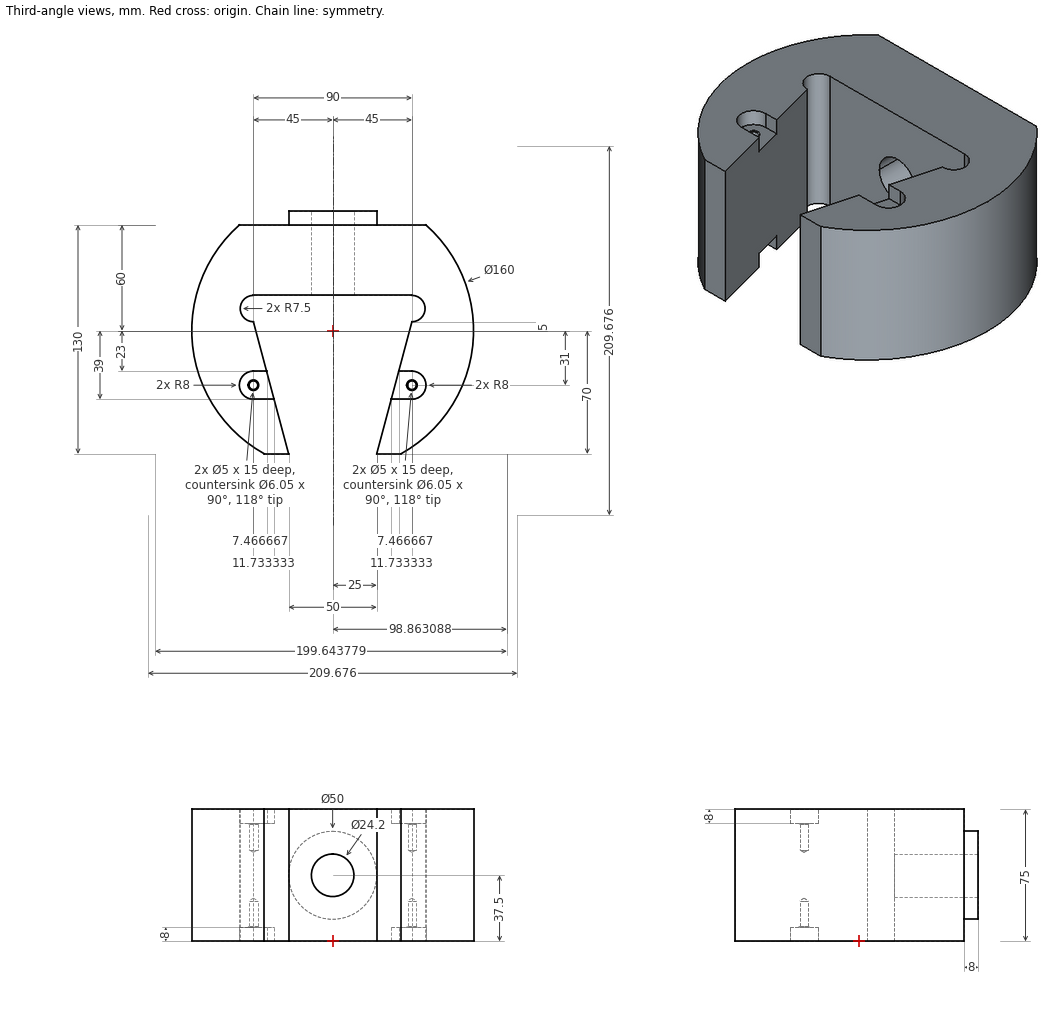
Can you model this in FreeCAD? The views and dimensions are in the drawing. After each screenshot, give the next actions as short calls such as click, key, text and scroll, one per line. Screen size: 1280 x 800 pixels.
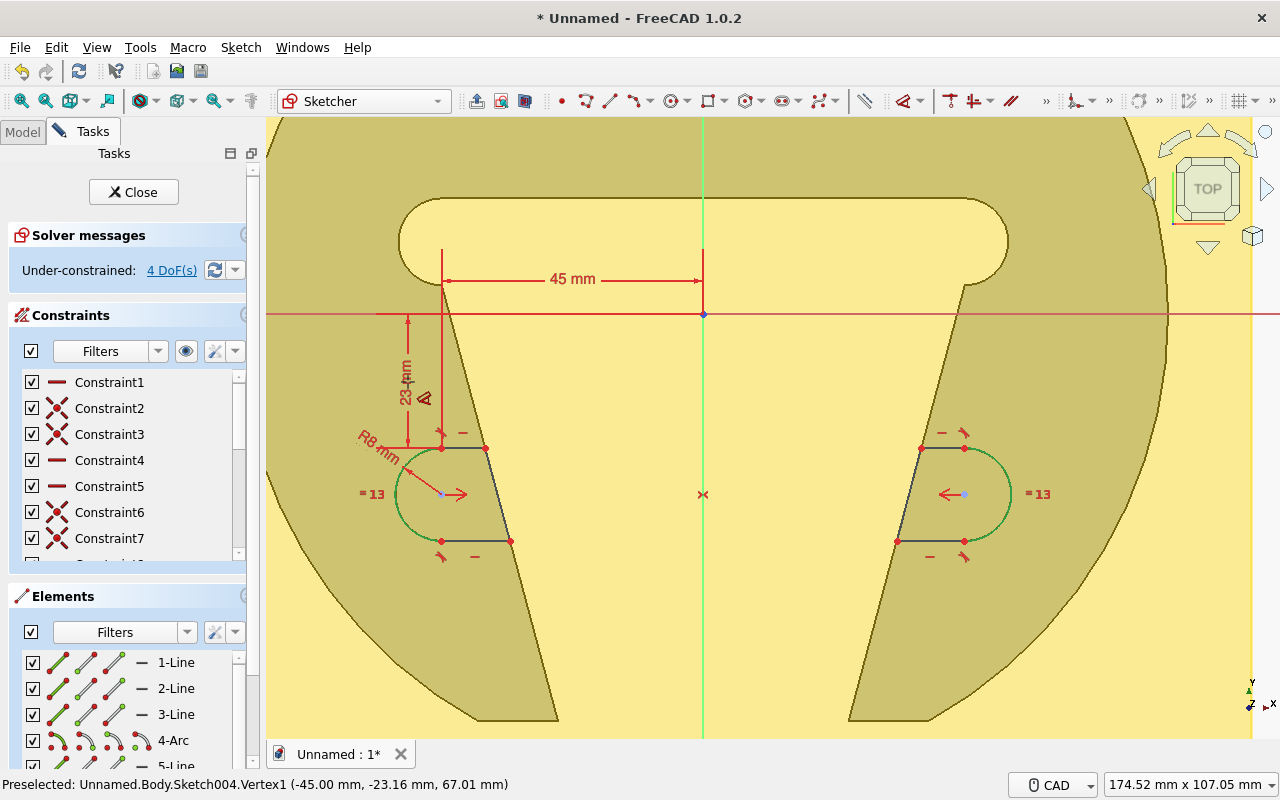
click(455, 448)
click(463, 482)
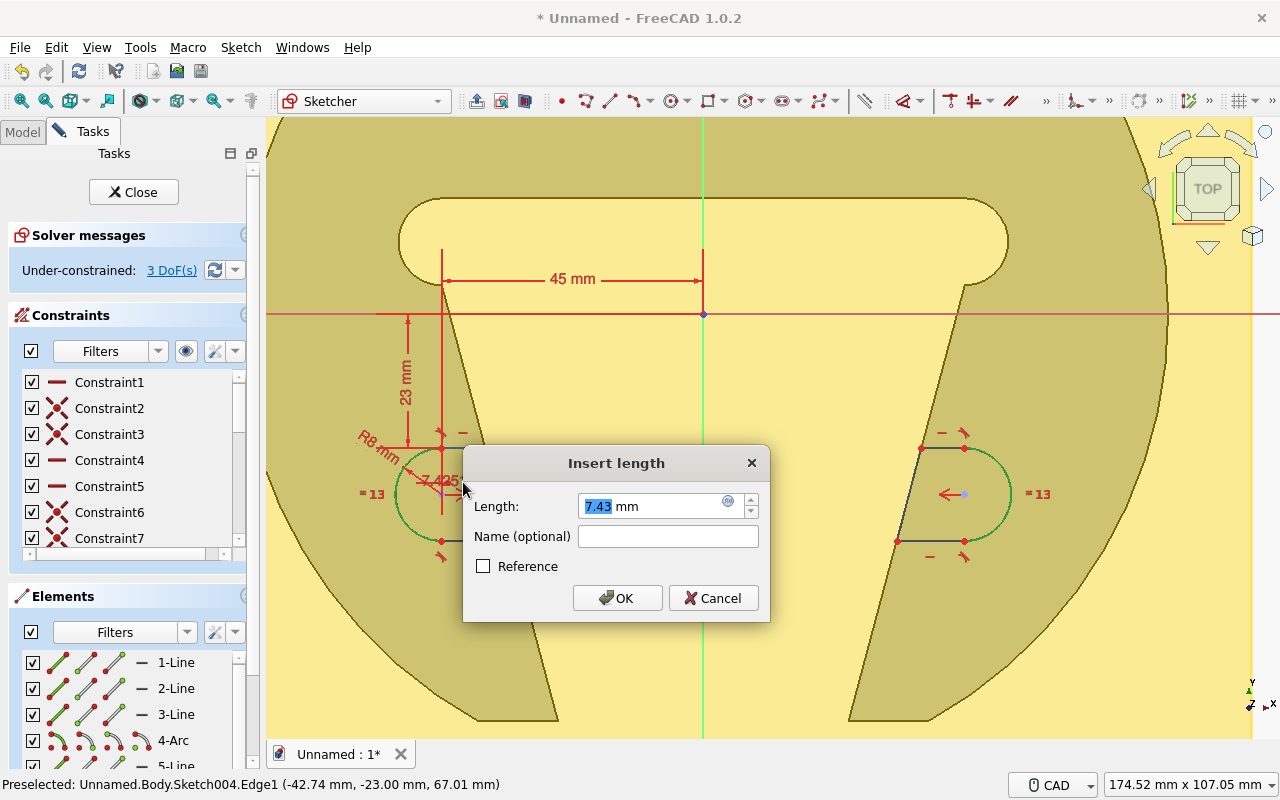
text(7.466667)
key(Return)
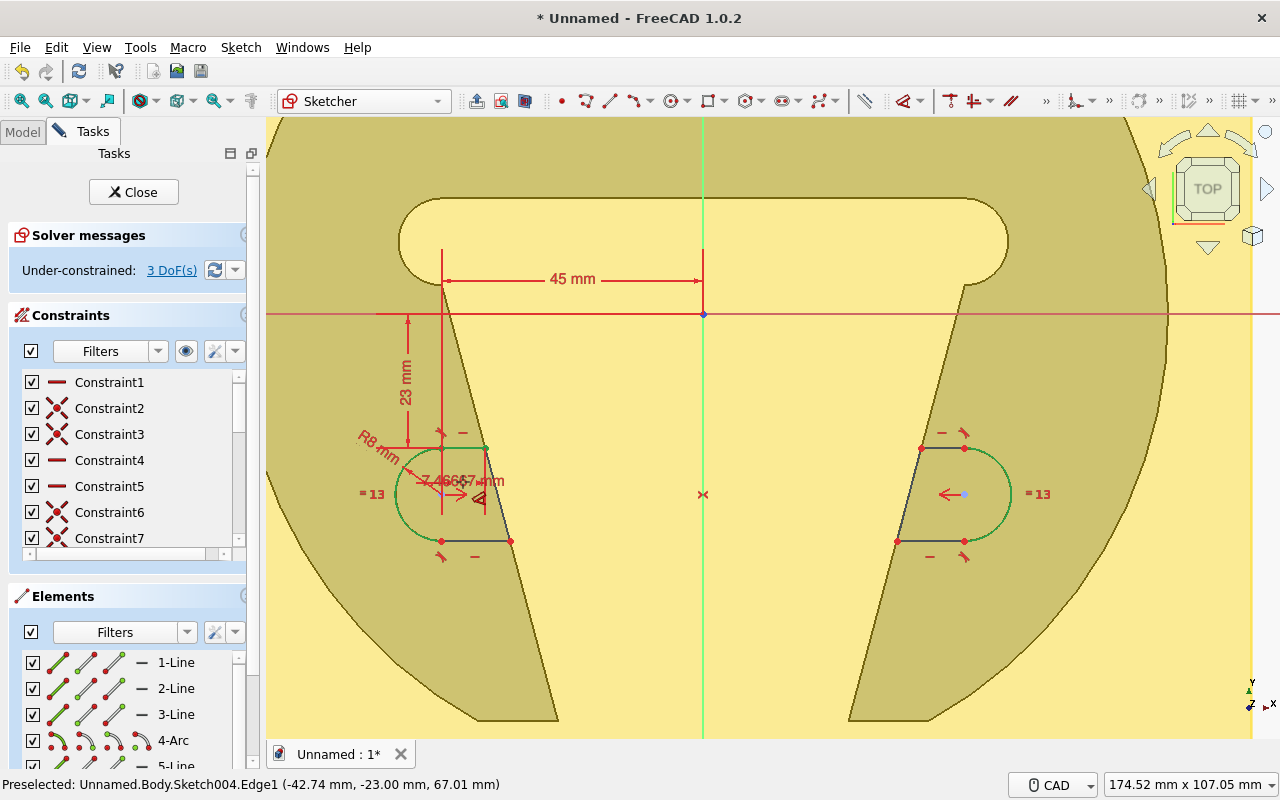
click(934, 448)
click(943, 482)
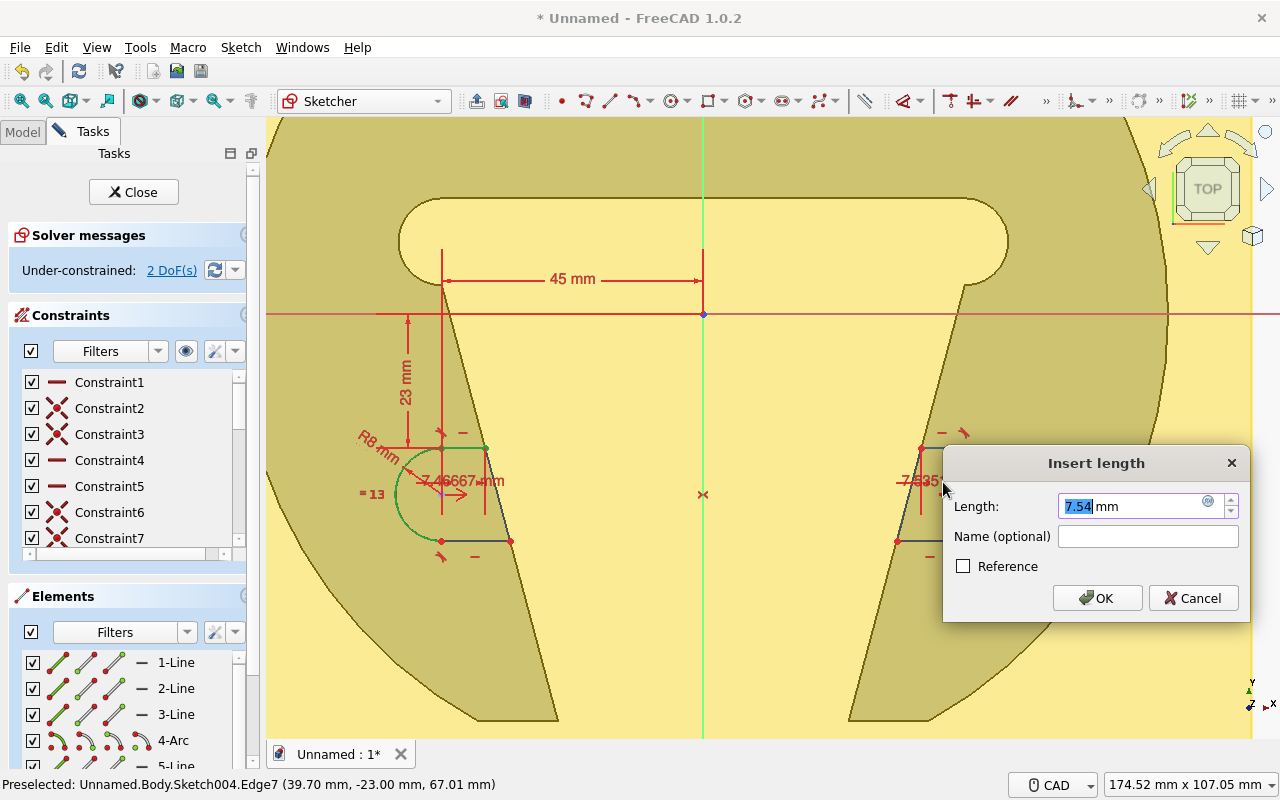
text(7.466667)
key(Return)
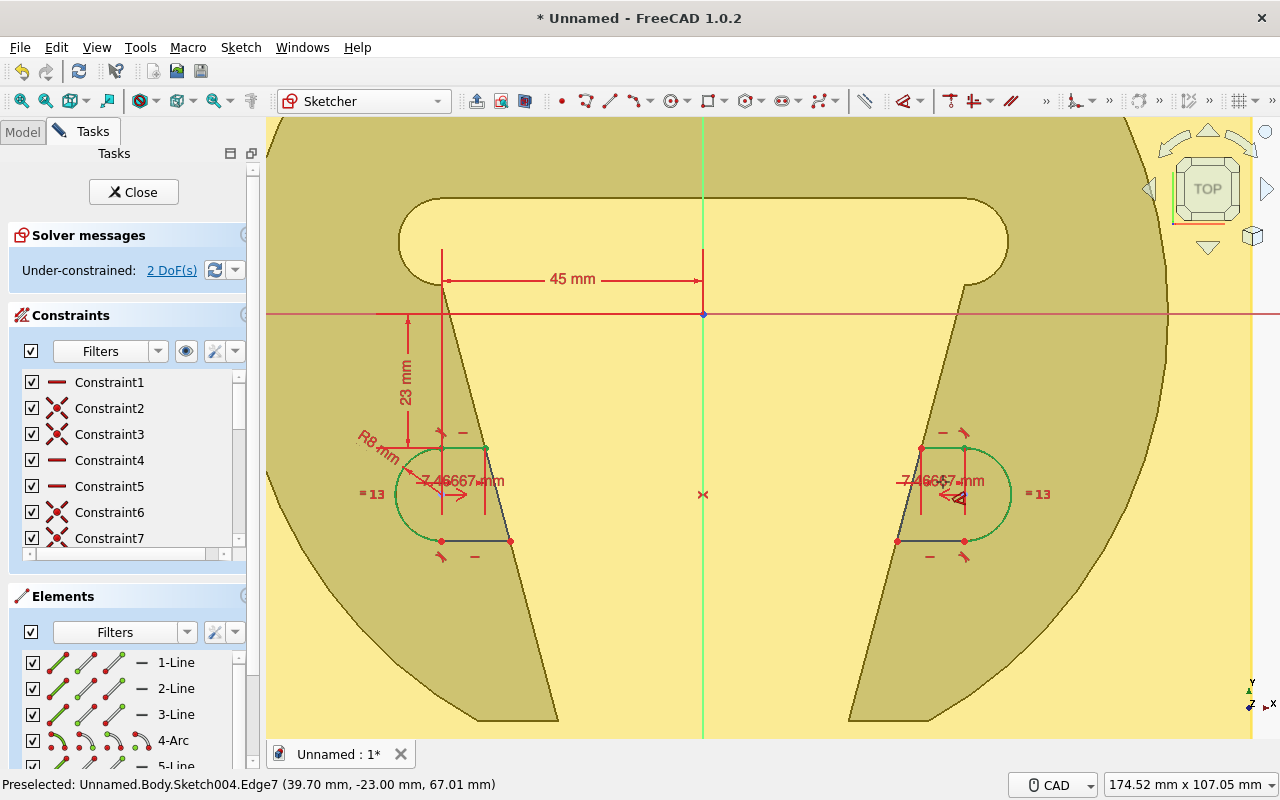
click(490, 541)
click(476, 575)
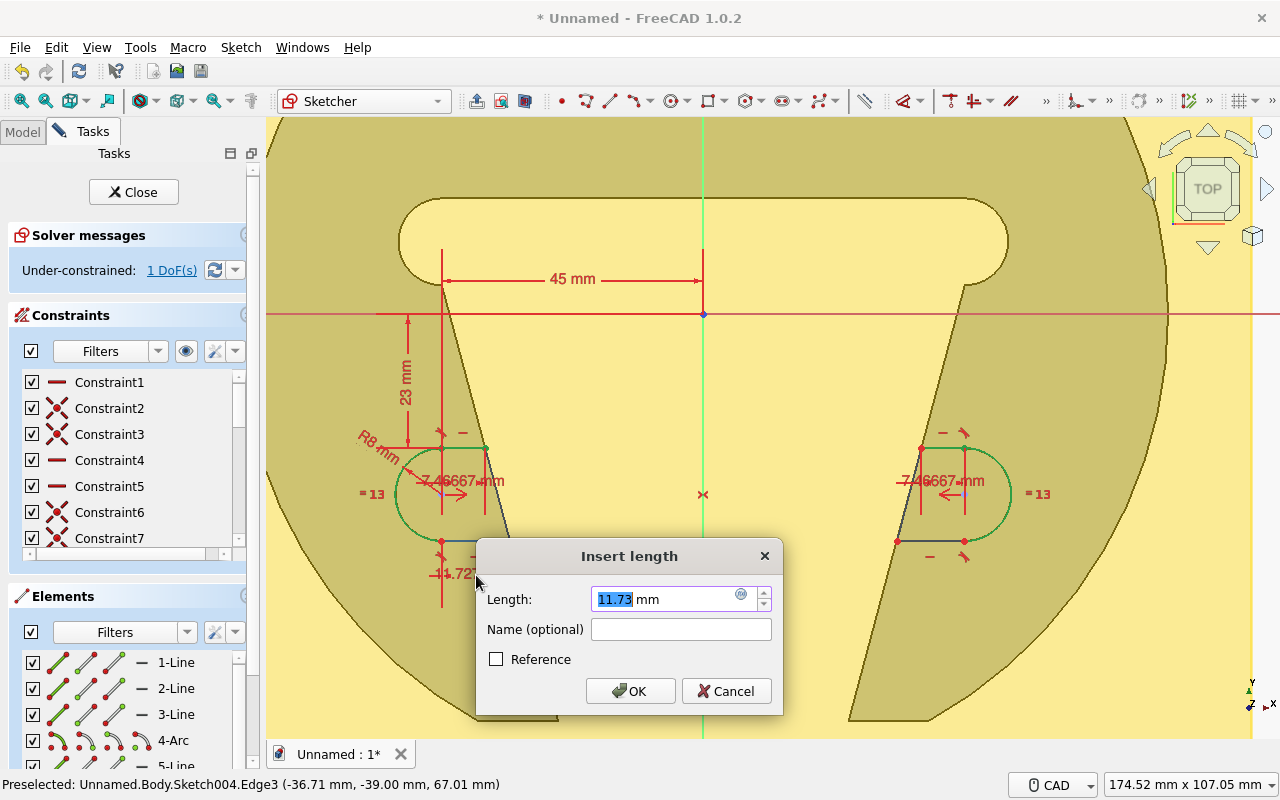
text(11.733333)
key(Return)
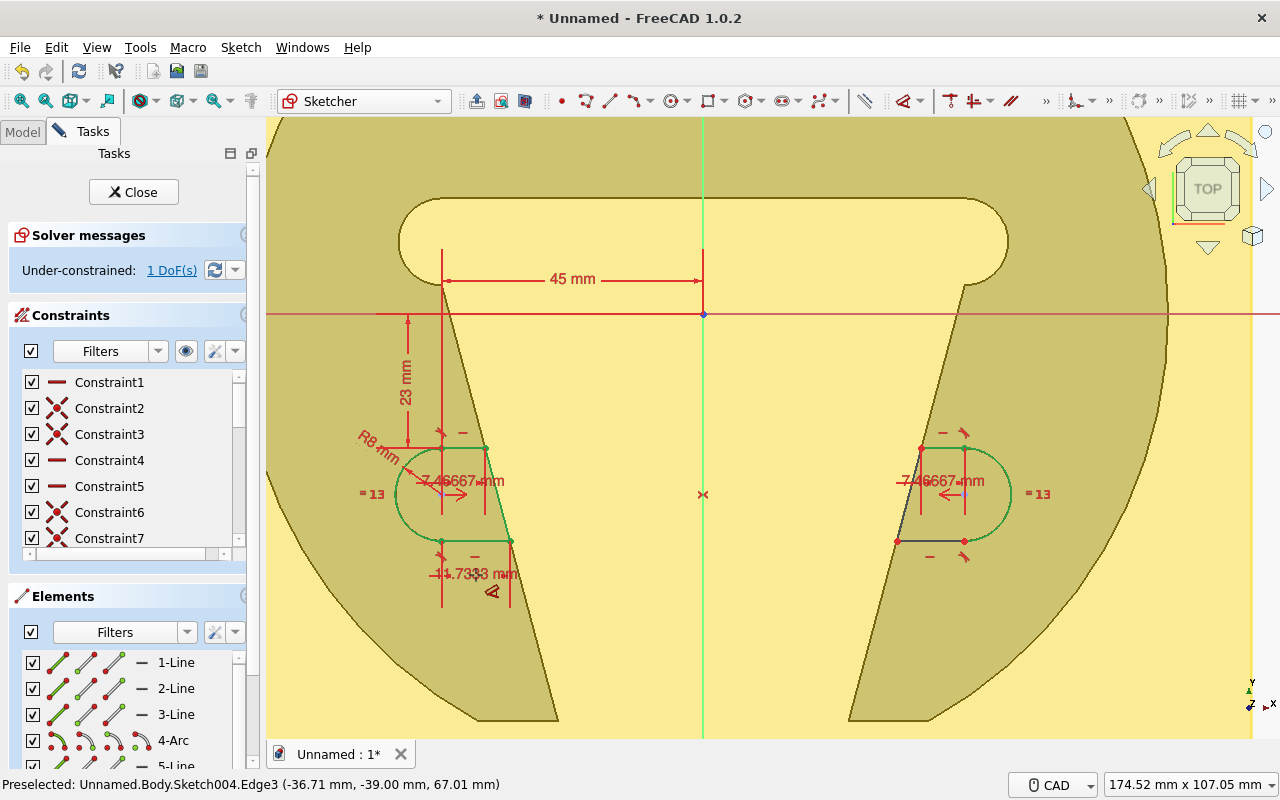
click(944, 541)
click(931, 575)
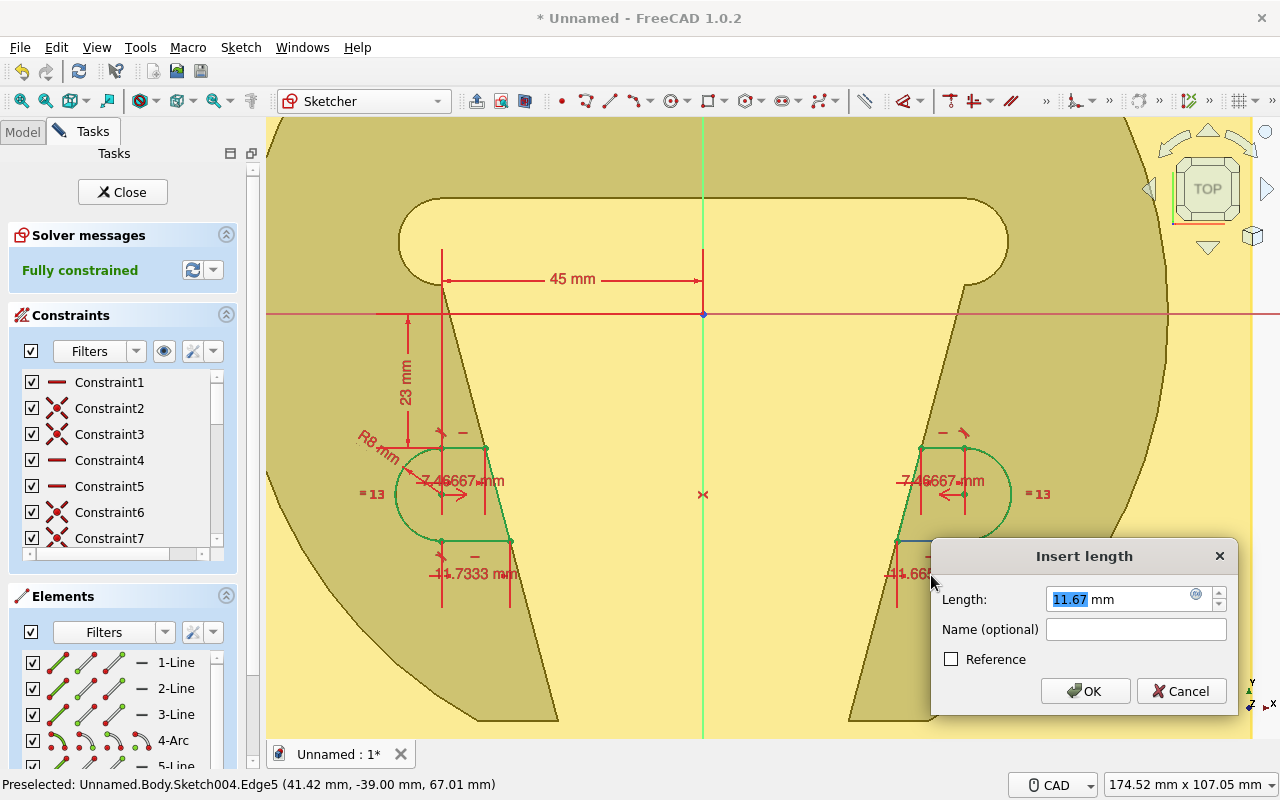
text(11.733333)
key(Return)
key(Escape)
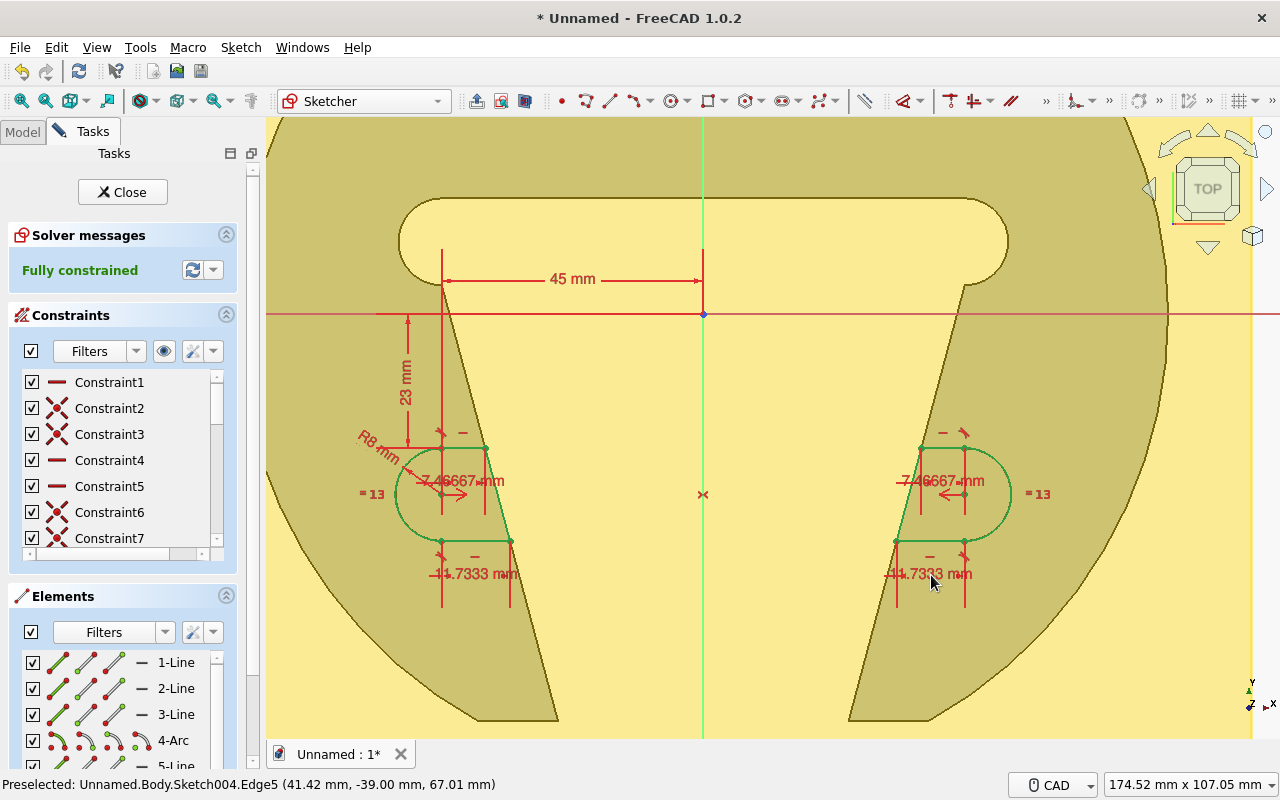
click(123, 192)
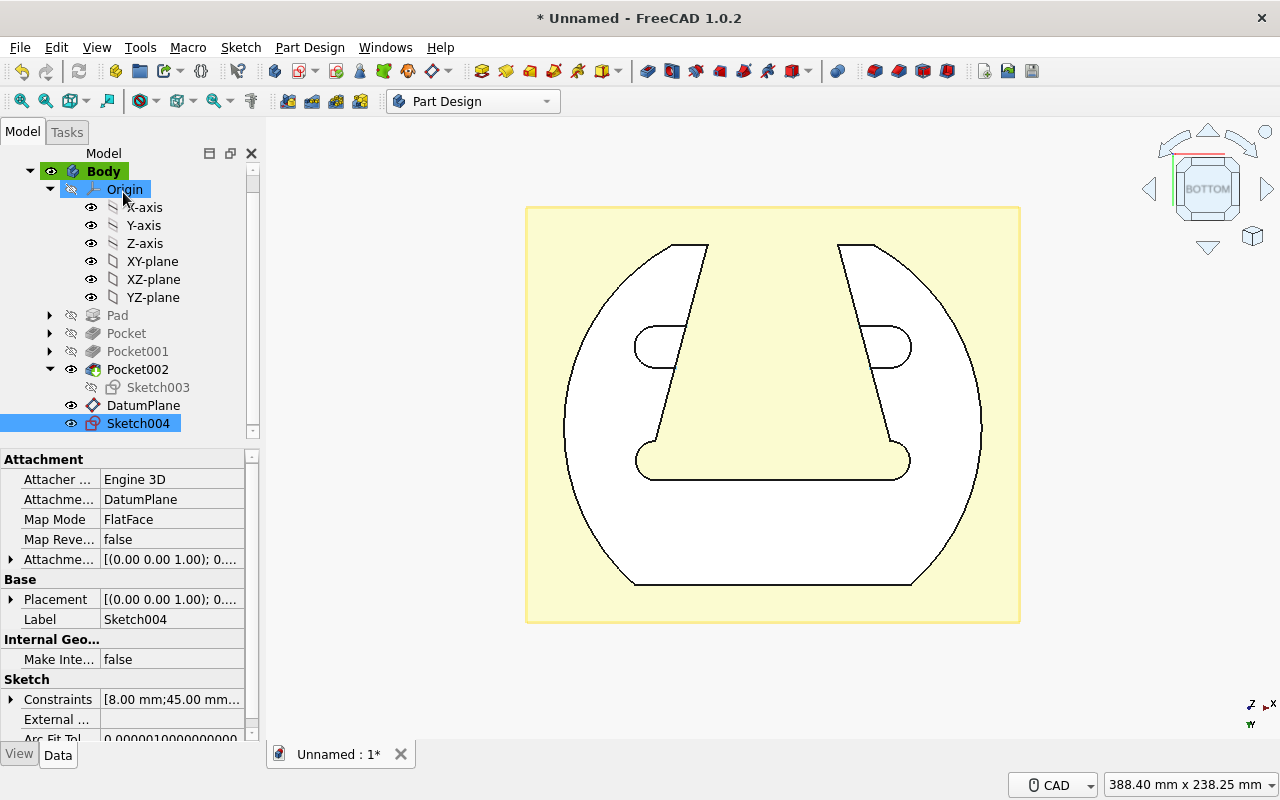
click(648, 72)